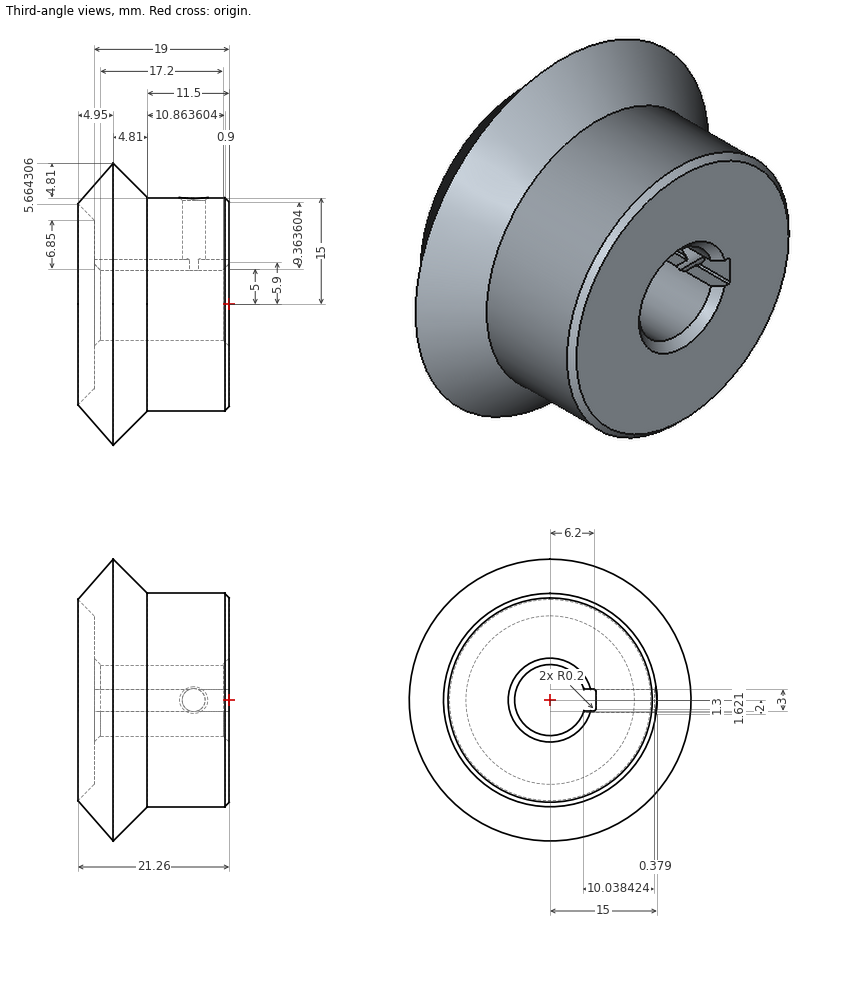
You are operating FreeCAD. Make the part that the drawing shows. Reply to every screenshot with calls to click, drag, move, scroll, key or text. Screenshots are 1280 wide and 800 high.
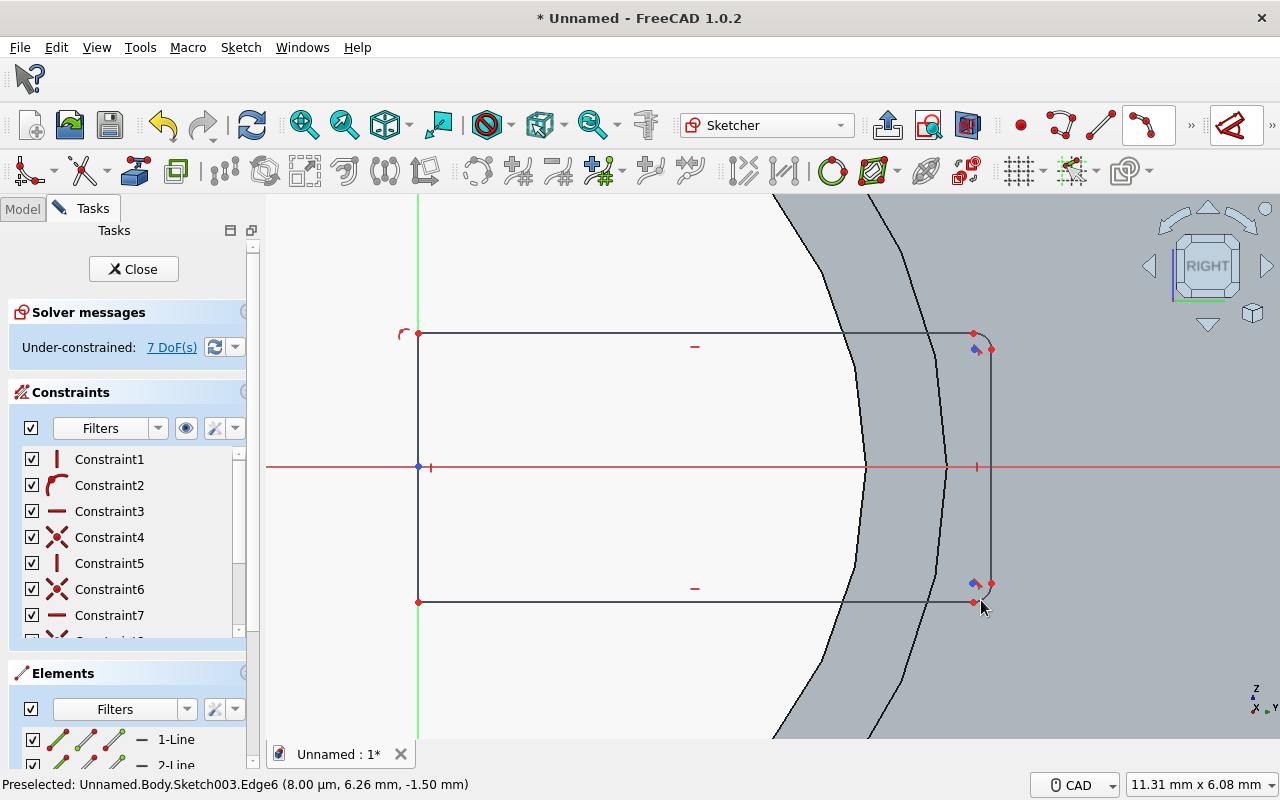
click(807, 333)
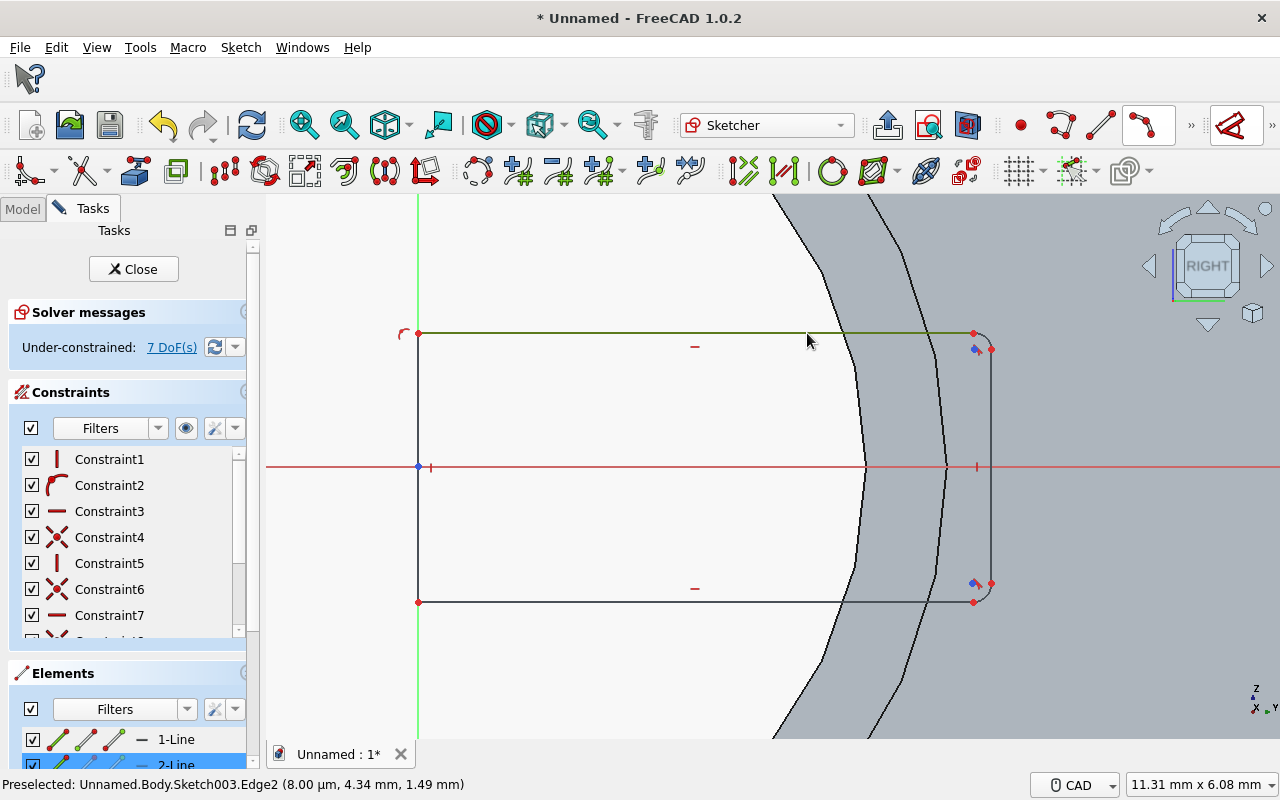
click(986, 338)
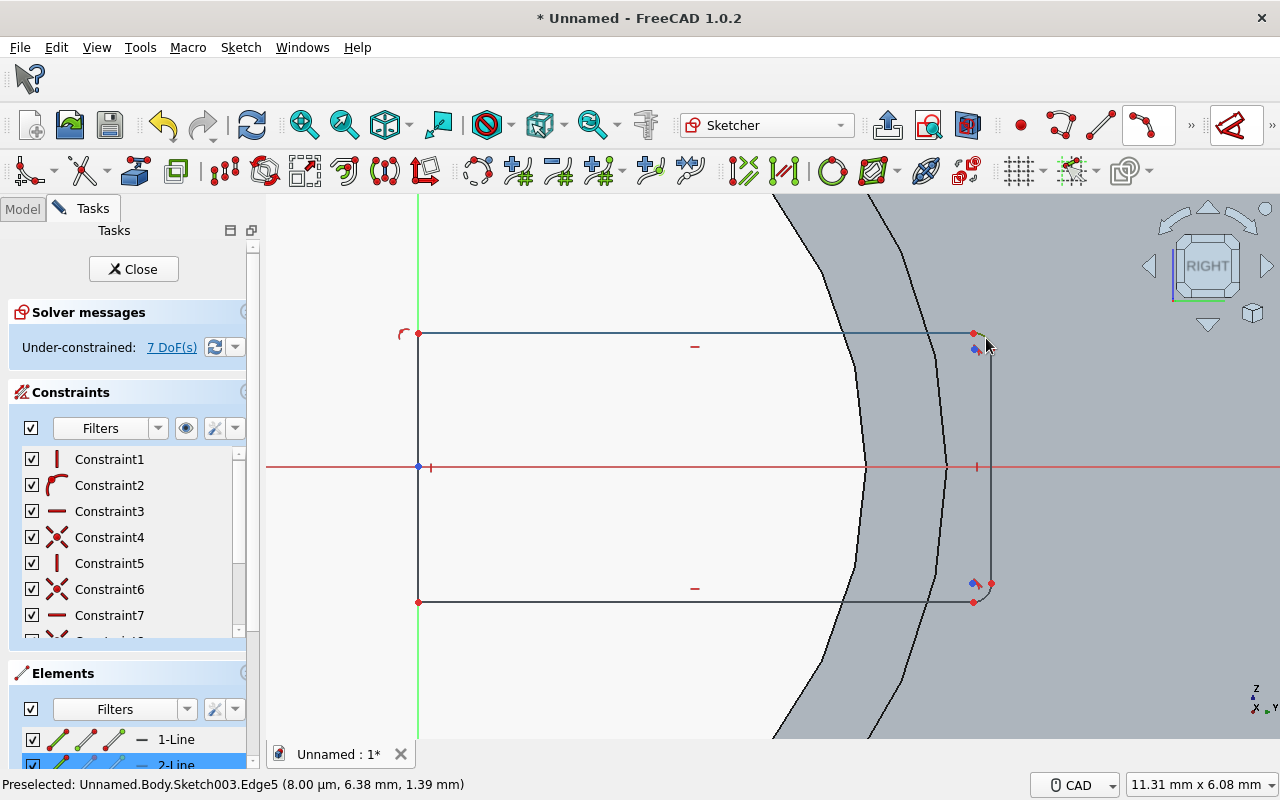
key(t)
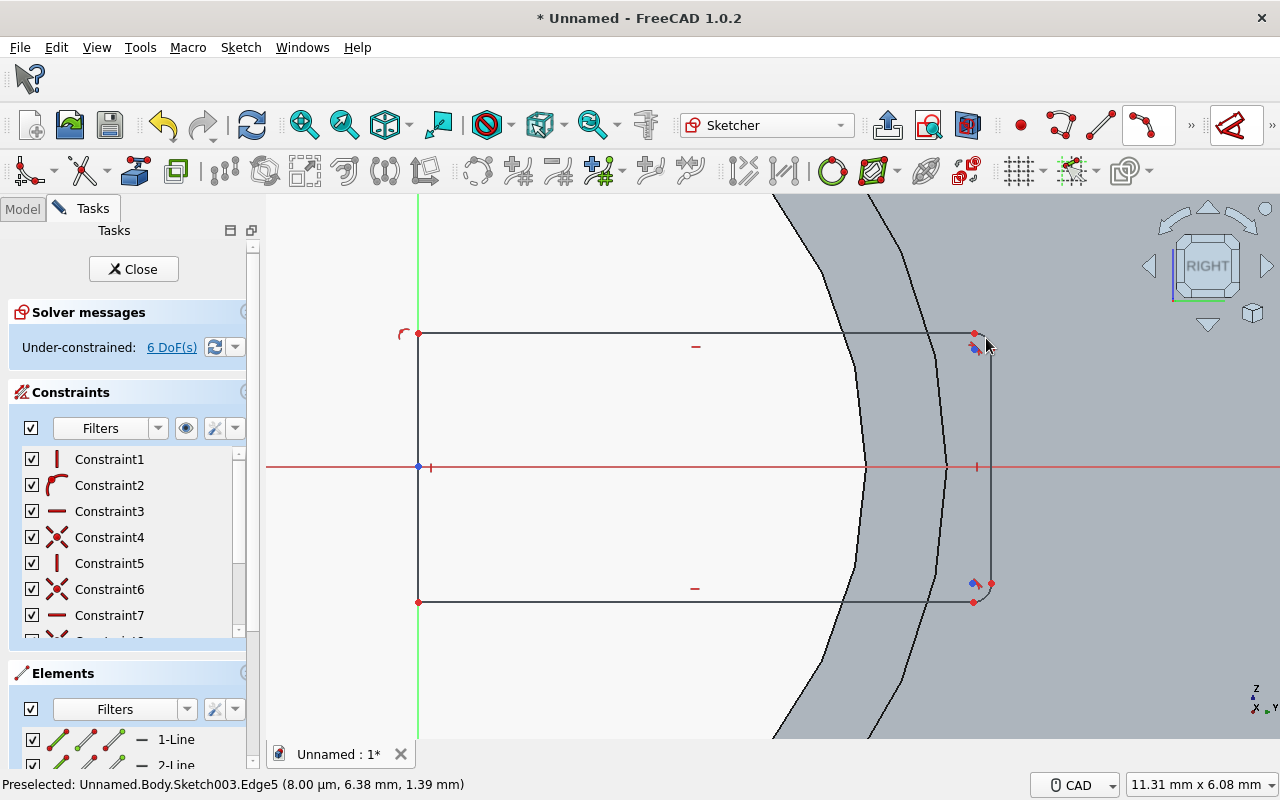
click(585, 602)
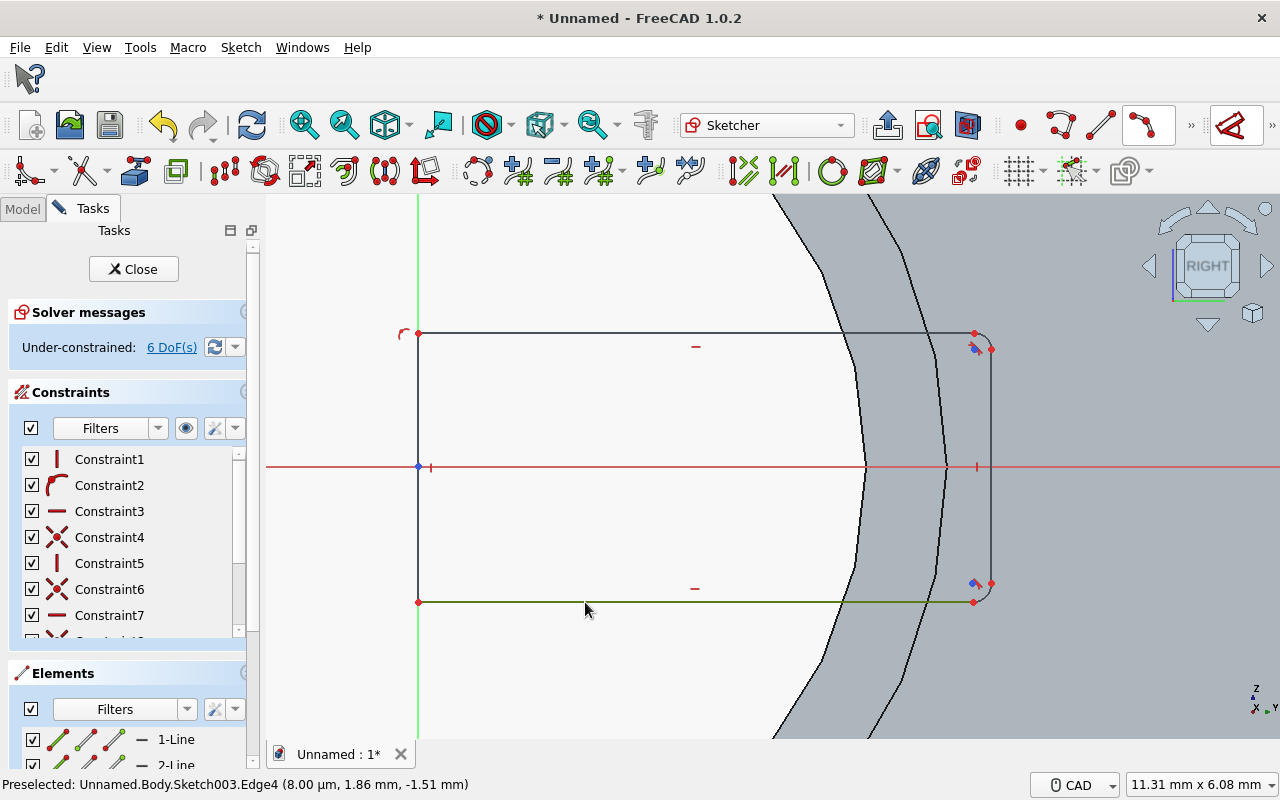
click(986, 597)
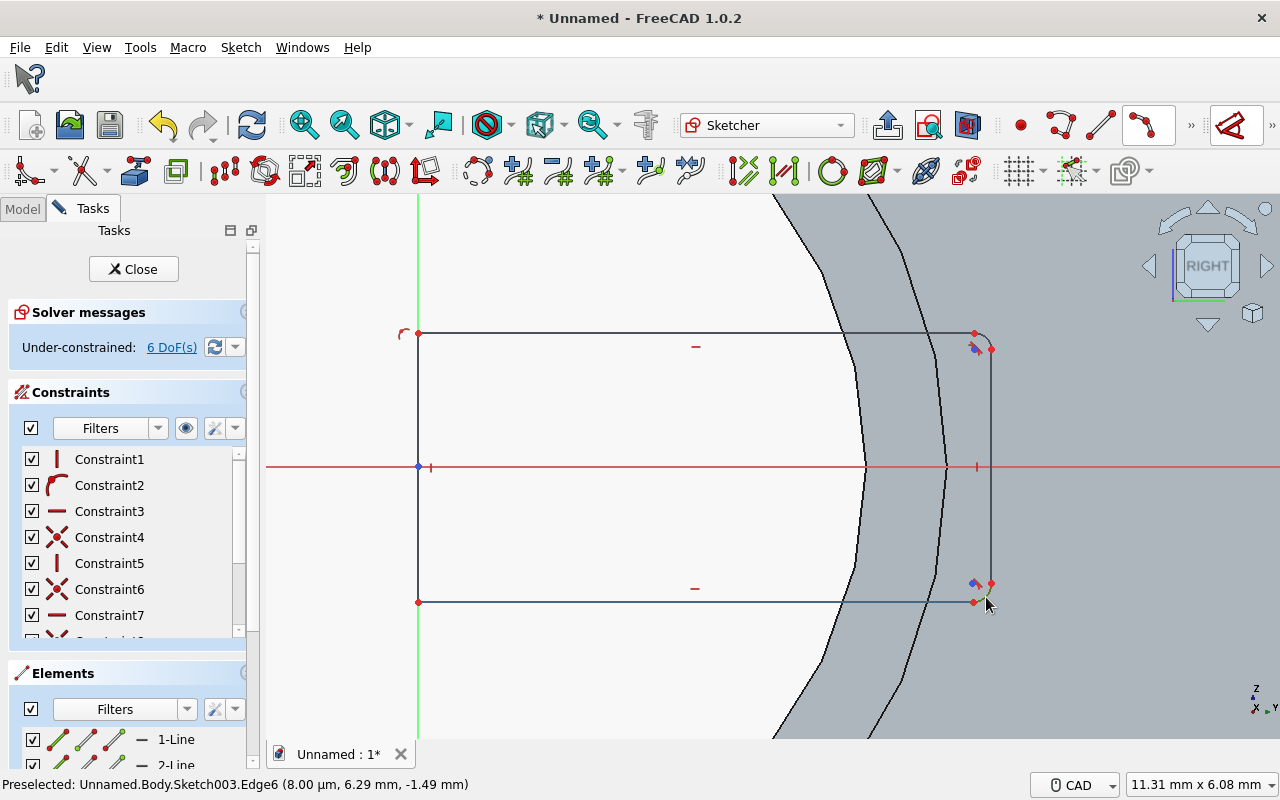
key(t)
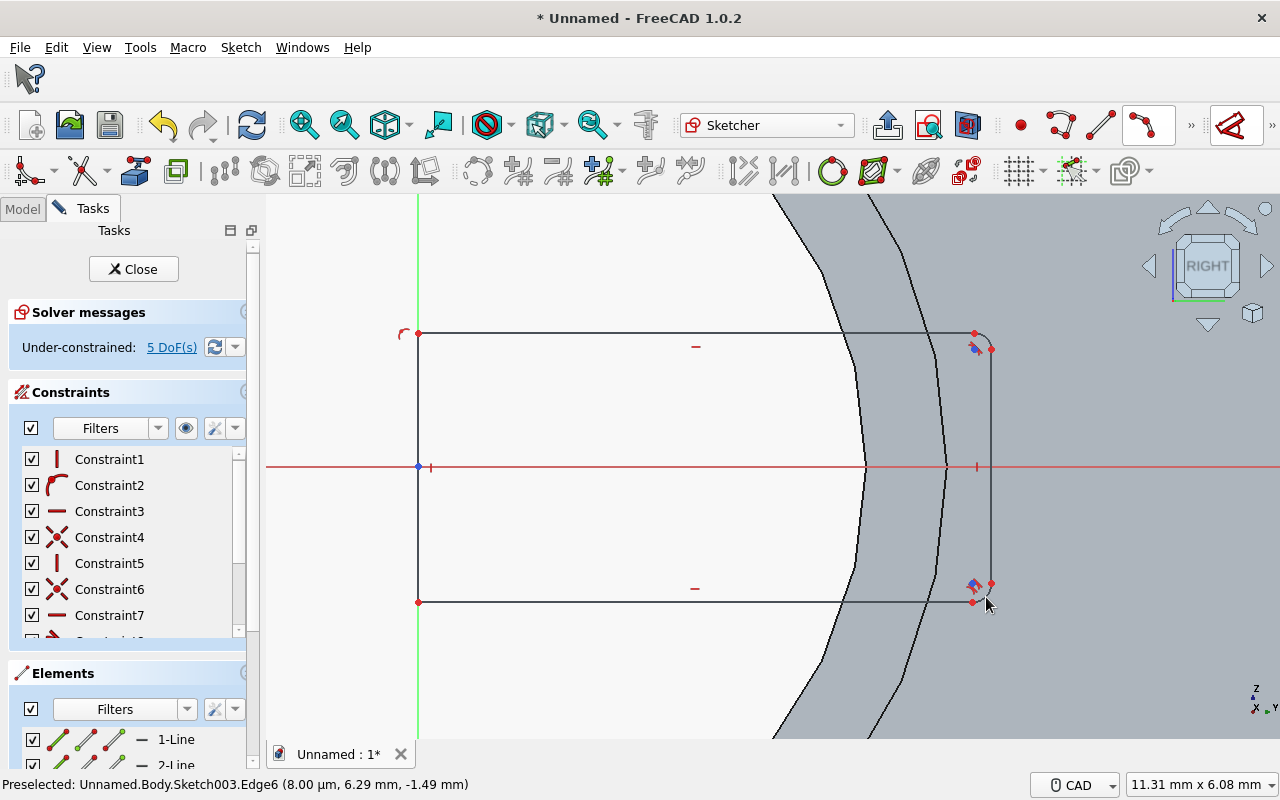
click(987, 338)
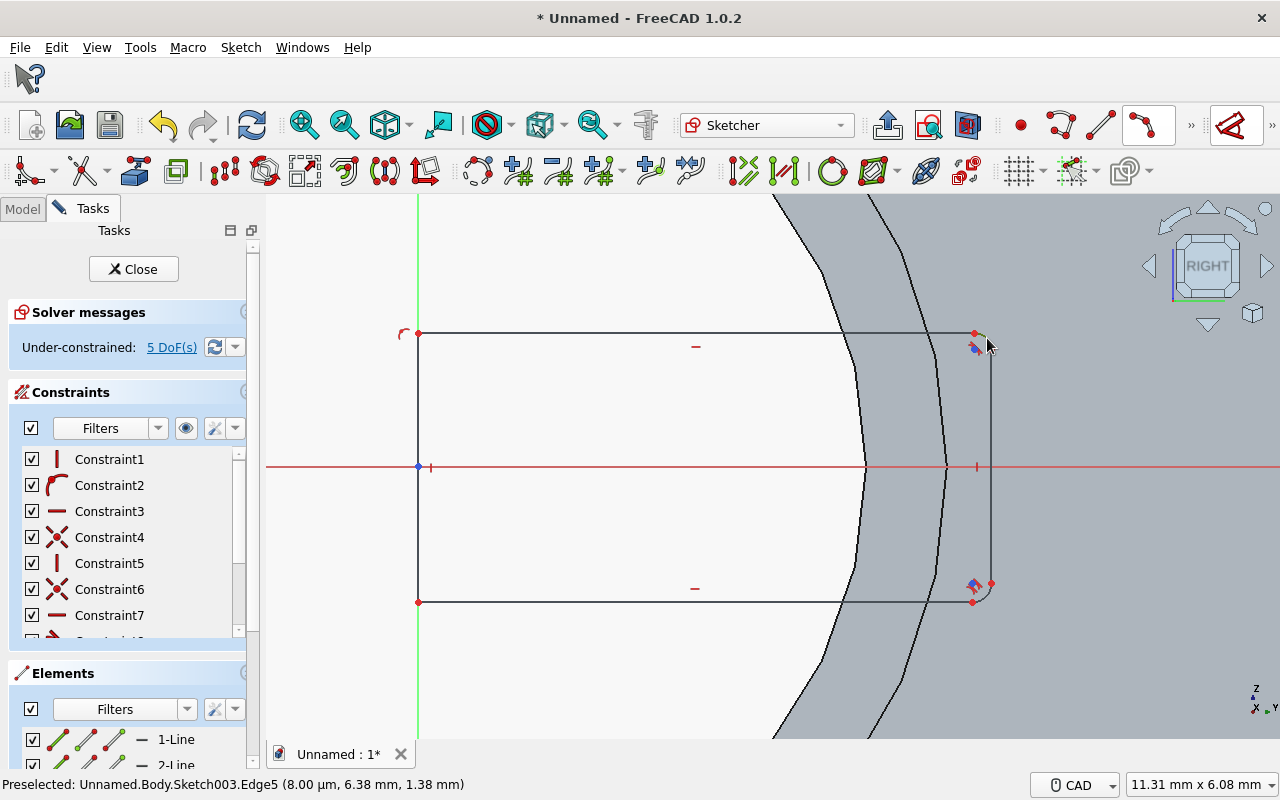
click(986, 597)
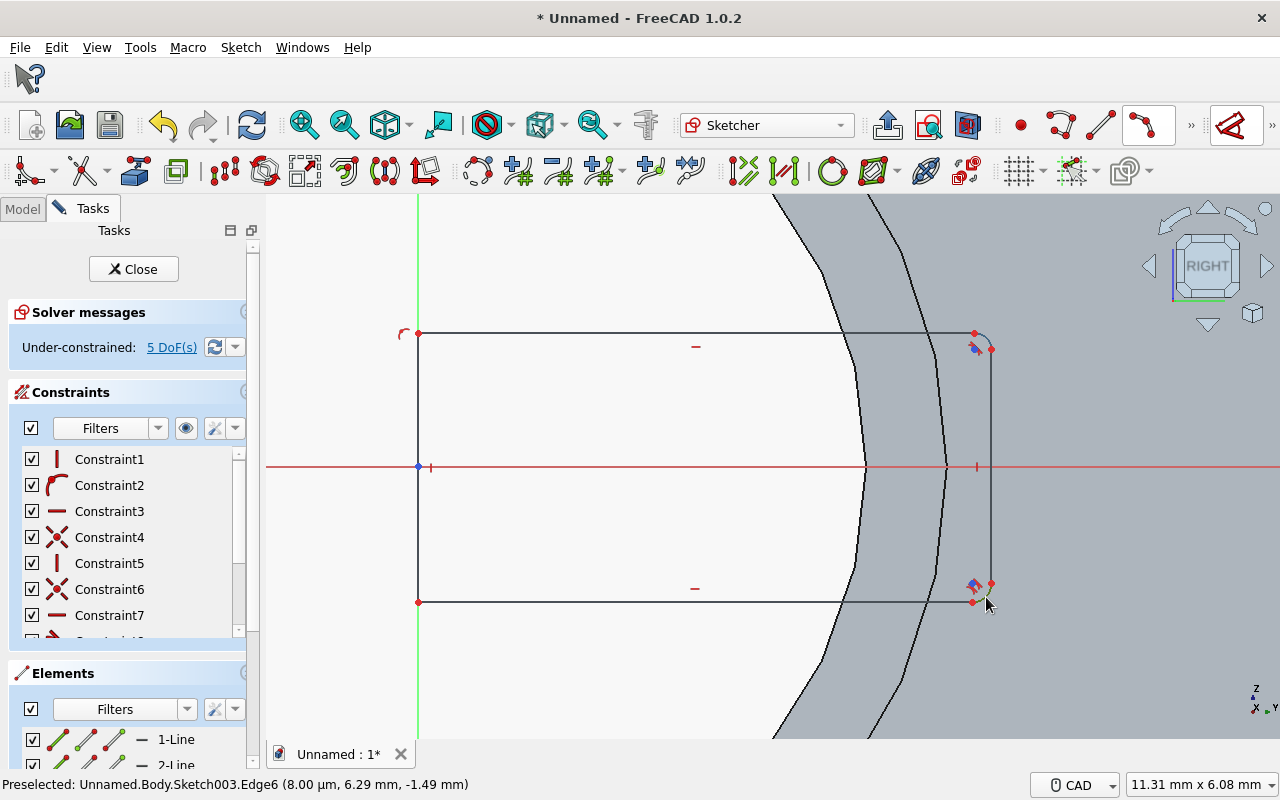
key(e)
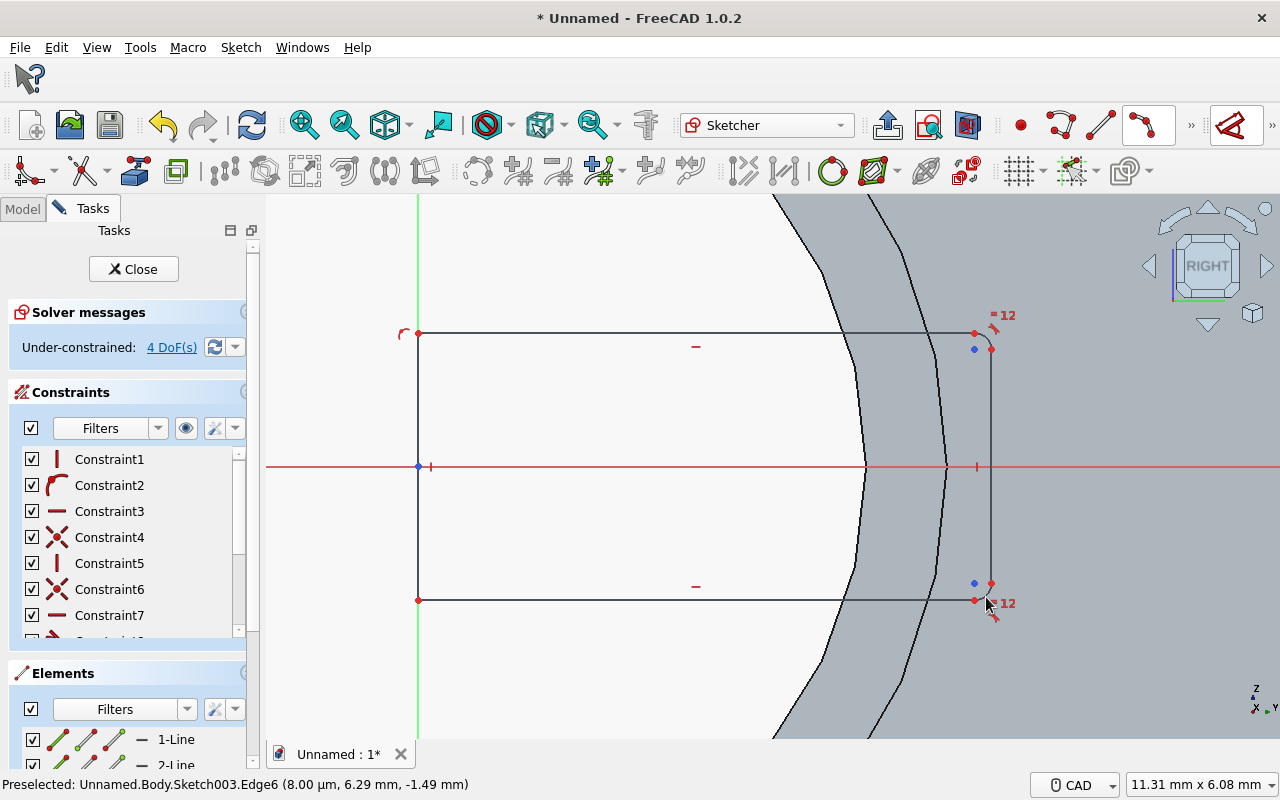
scroll(987, 338, up, 4)